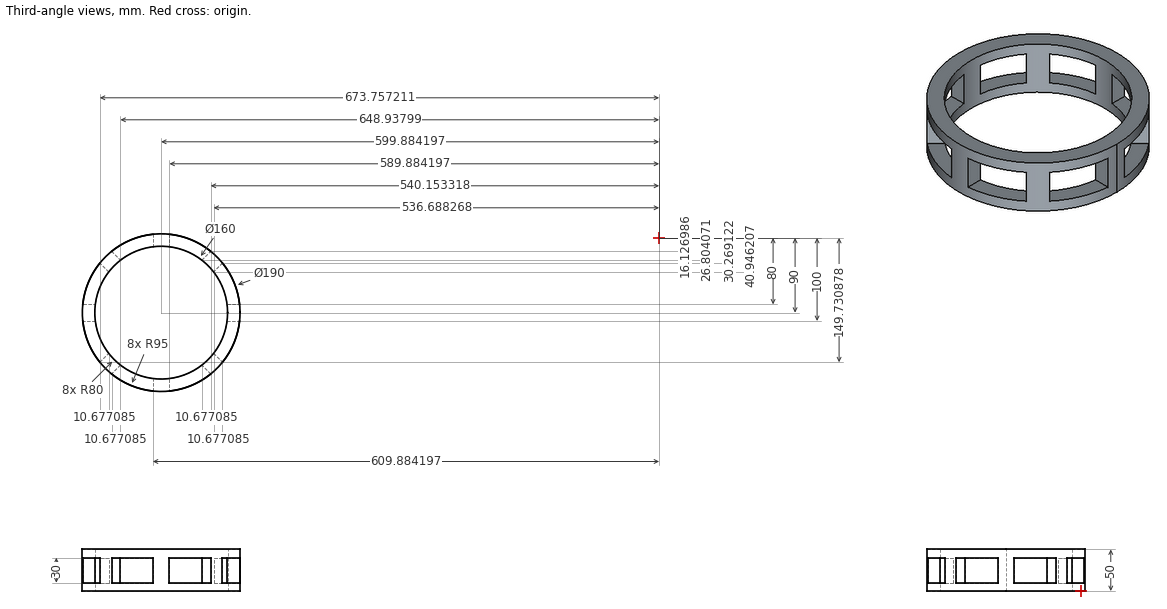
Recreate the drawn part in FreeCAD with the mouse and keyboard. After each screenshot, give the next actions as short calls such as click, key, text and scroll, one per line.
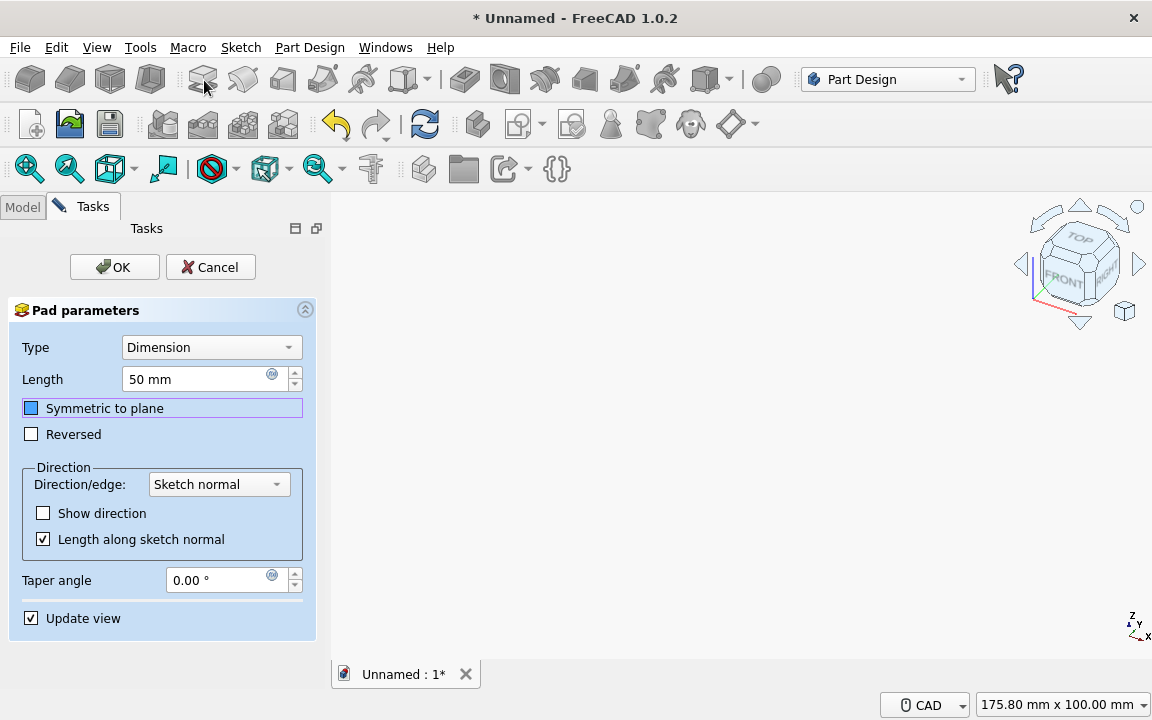
click(115, 267)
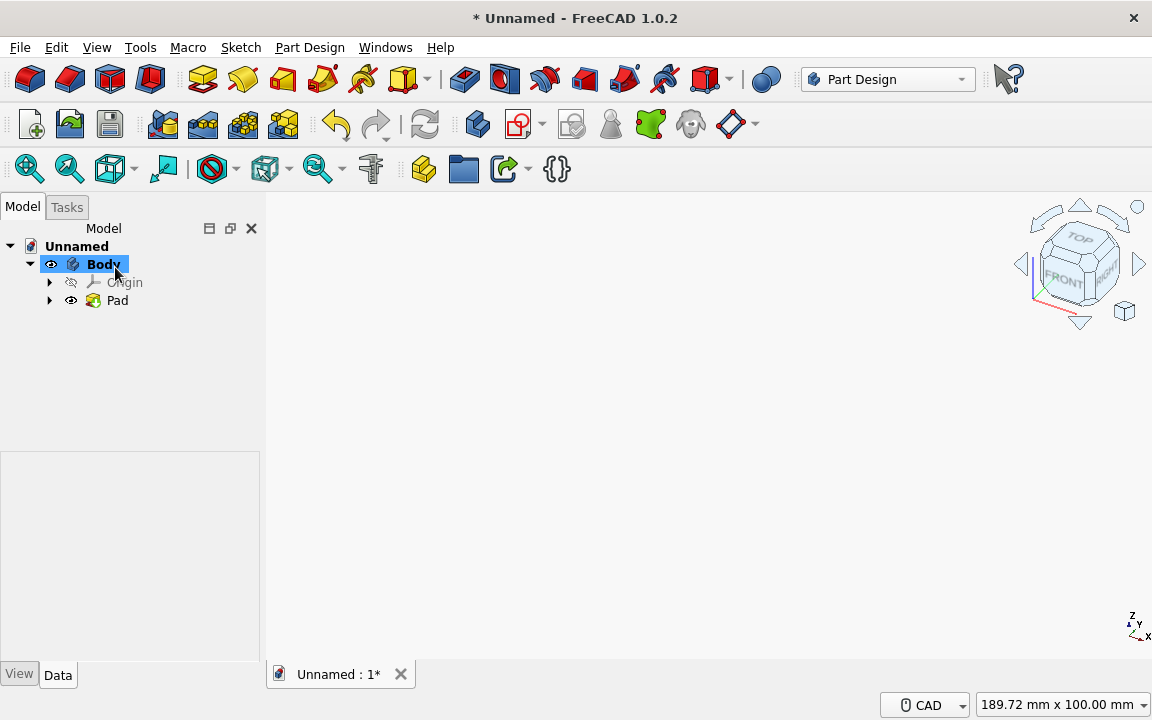
key(v)
key(f)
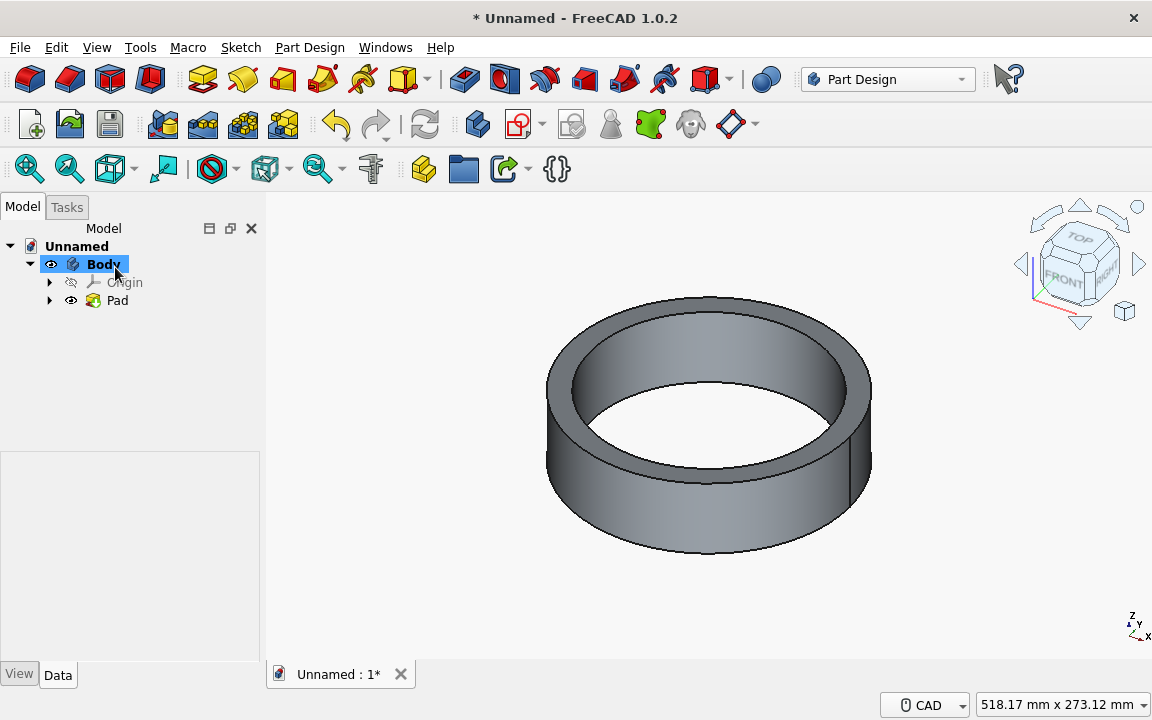
click(50, 282)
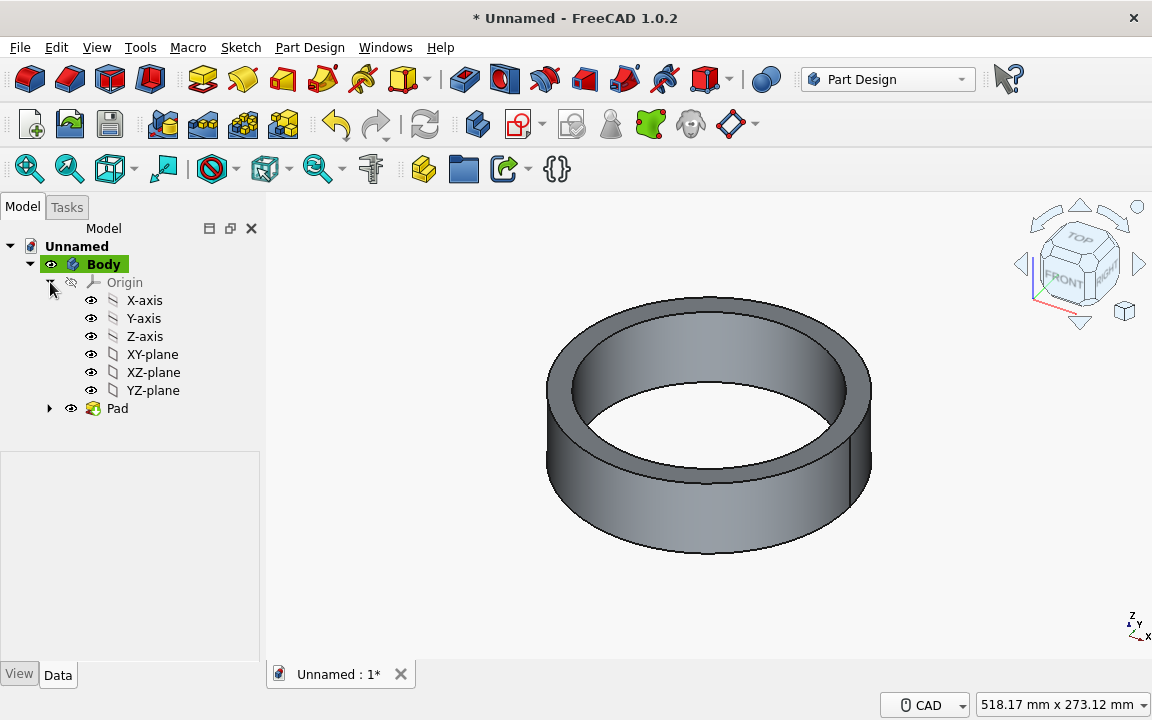
click(136, 354)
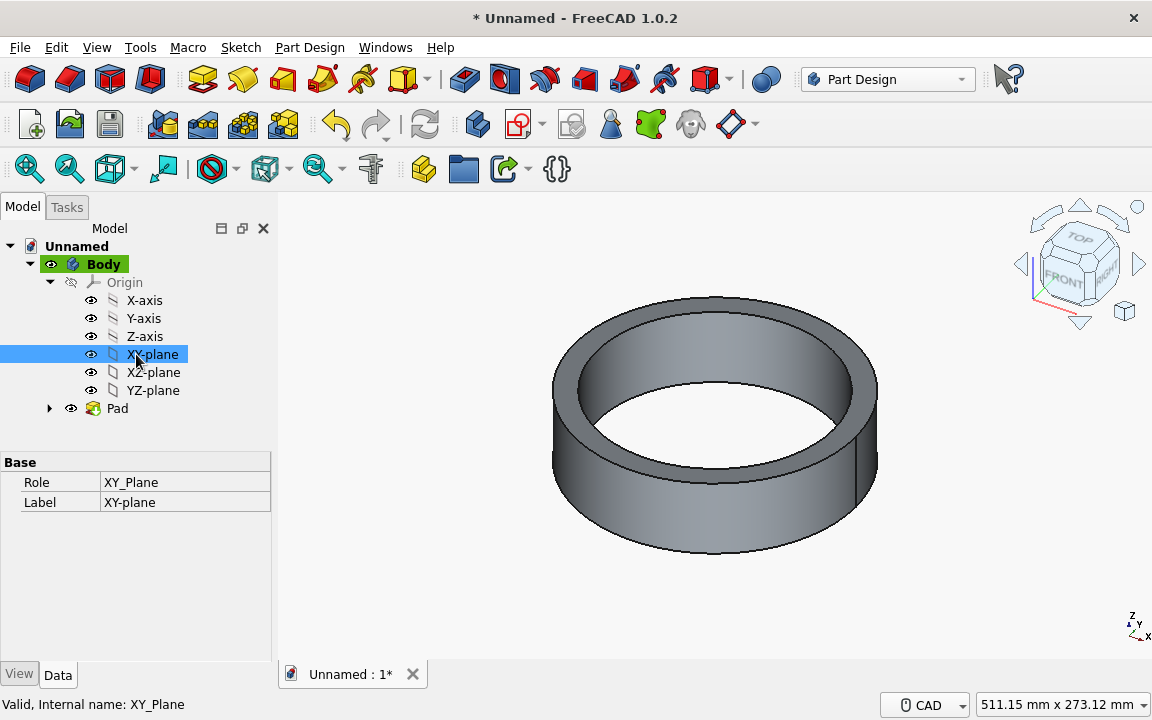
click(732, 124)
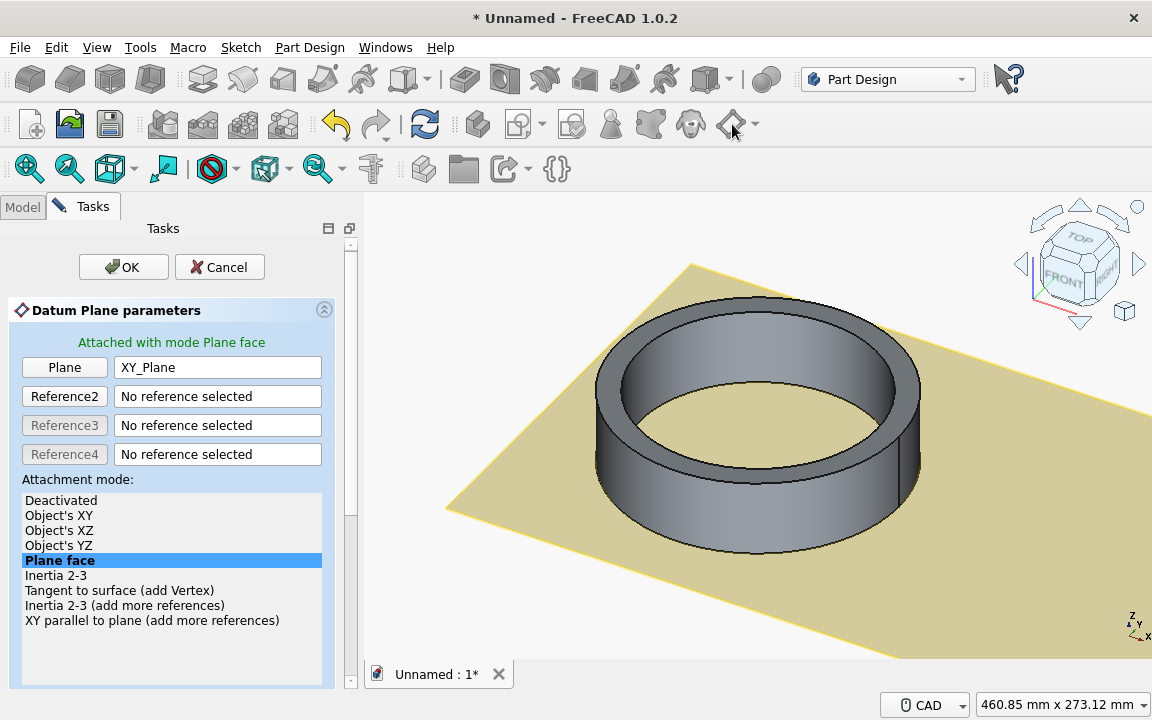
scroll(351, 463, down, 3)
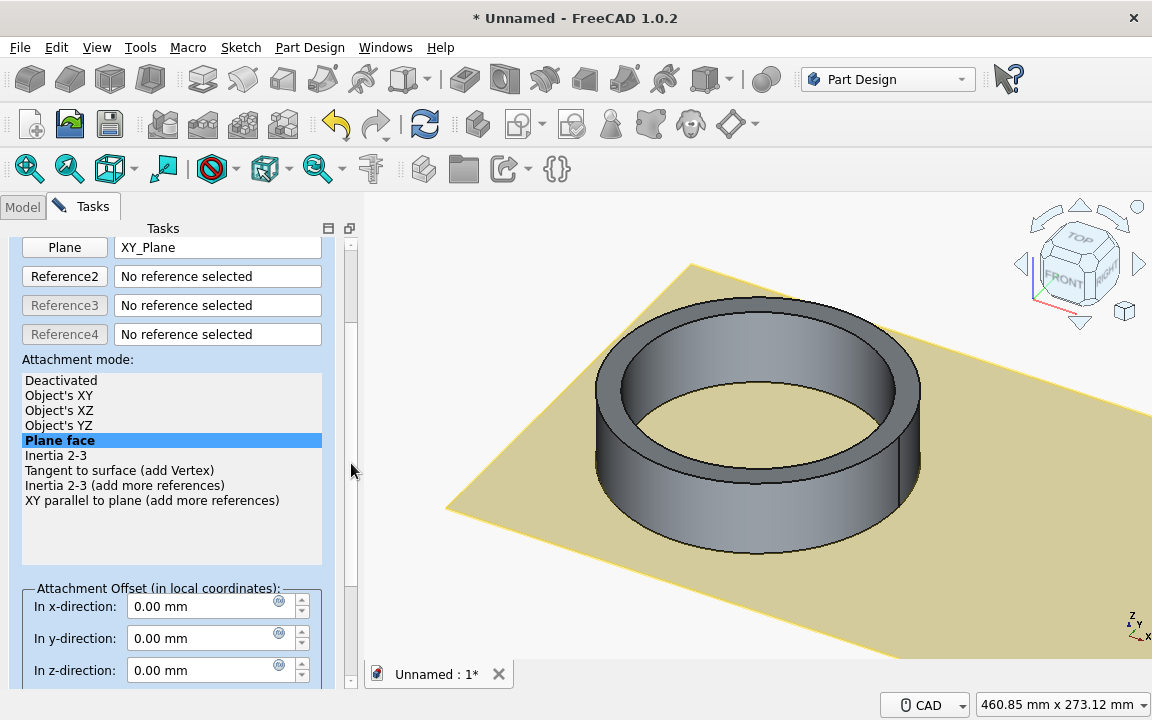
triple_click(210, 610)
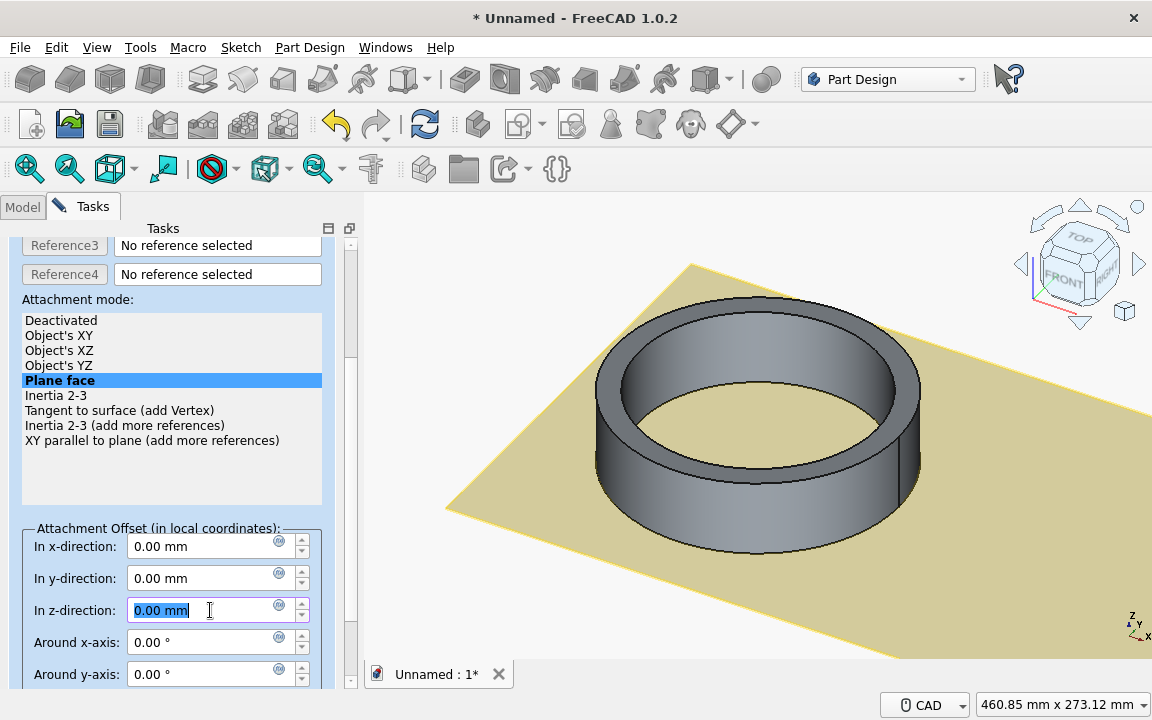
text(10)
key(Tab)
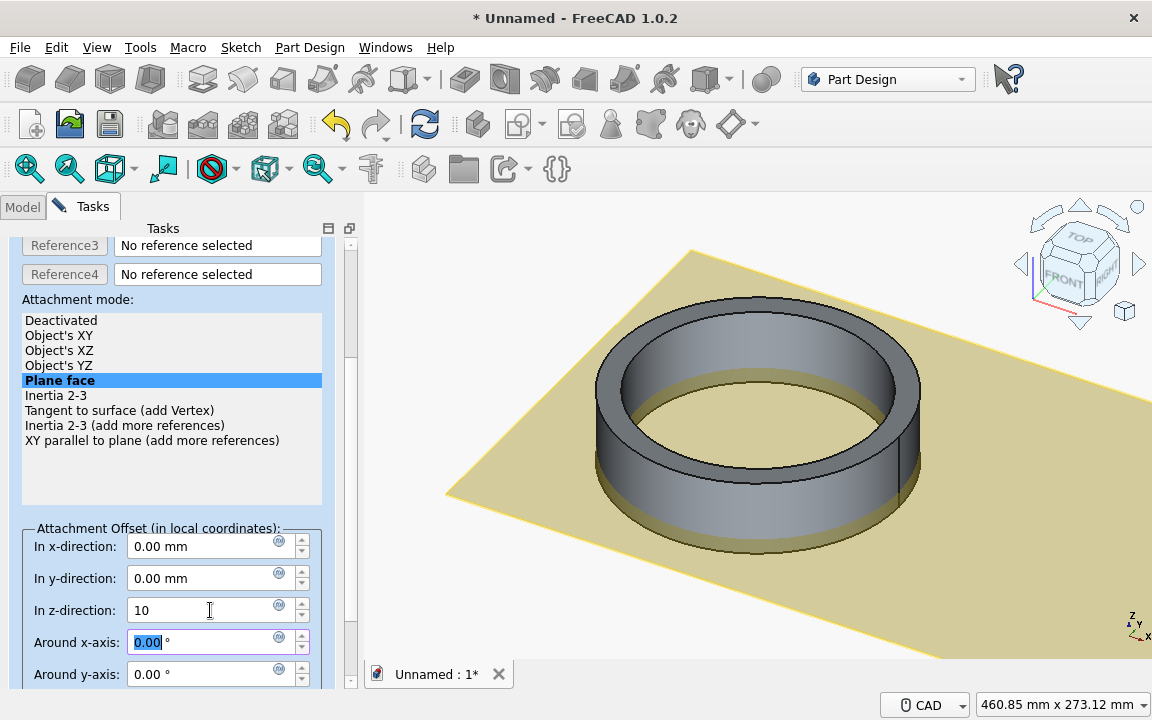
scroll(351, 463, up, 4)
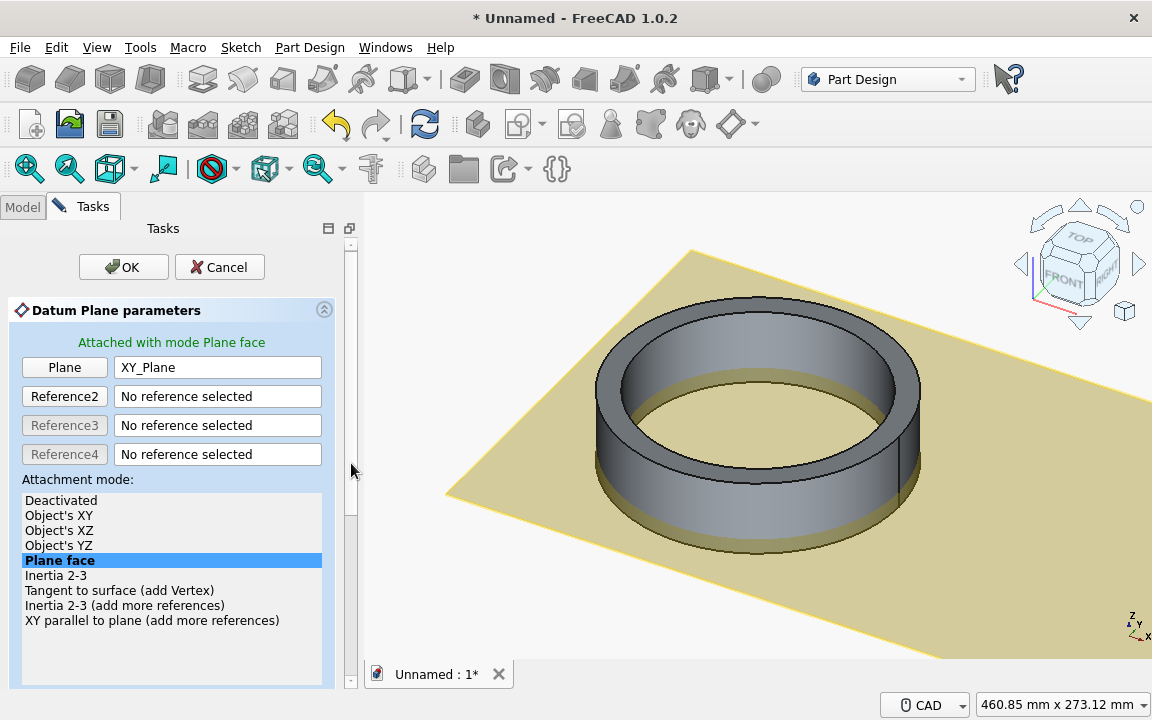
click(124, 267)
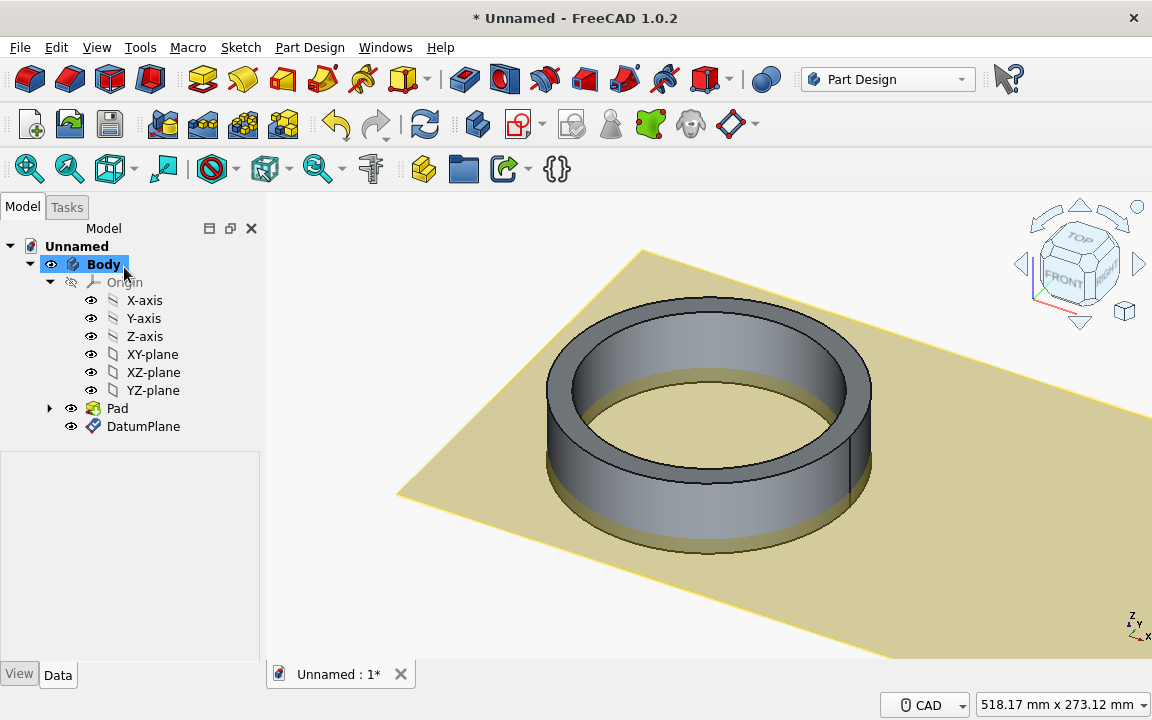
click(116, 426)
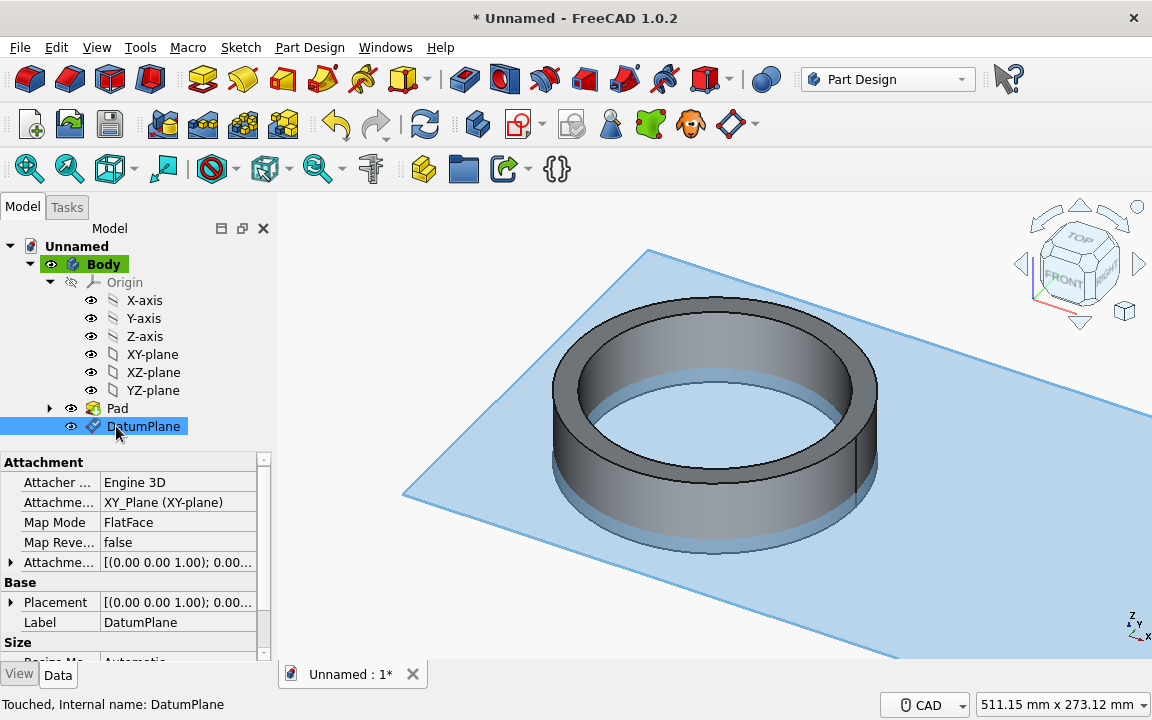
click(518, 124)